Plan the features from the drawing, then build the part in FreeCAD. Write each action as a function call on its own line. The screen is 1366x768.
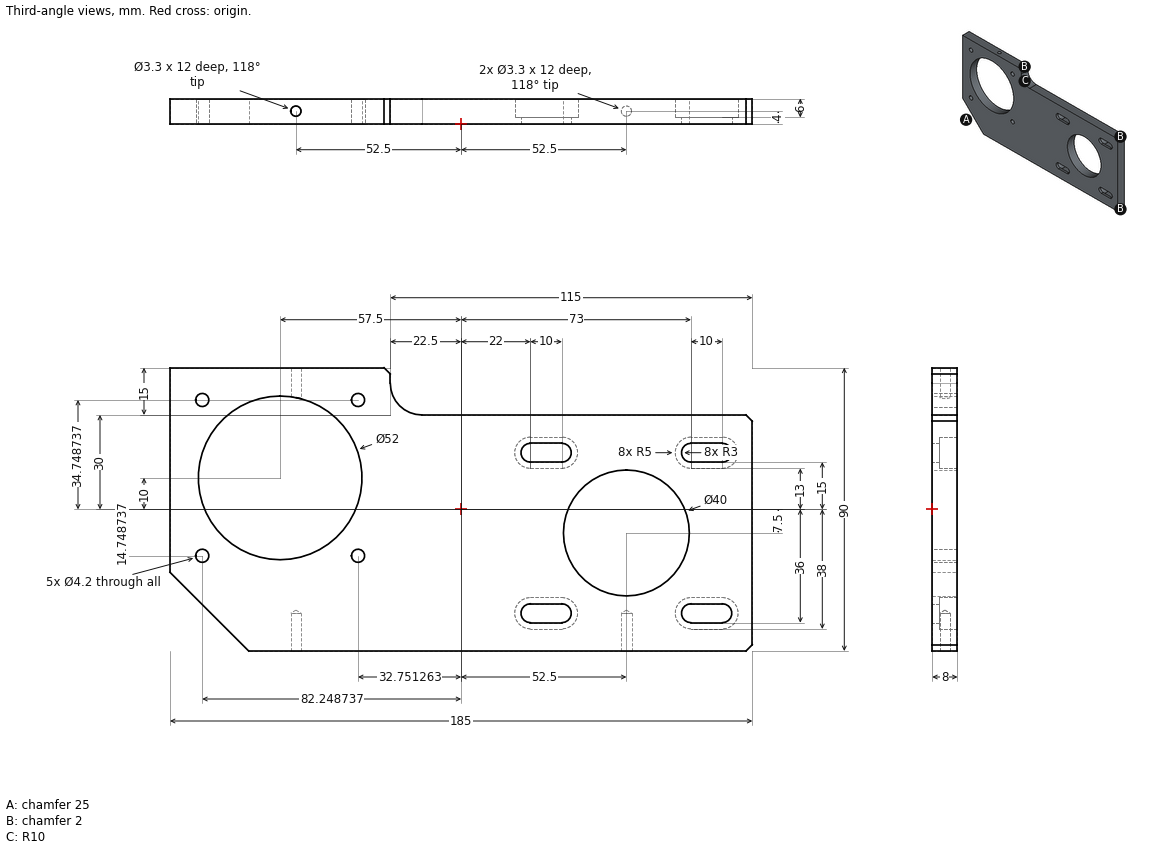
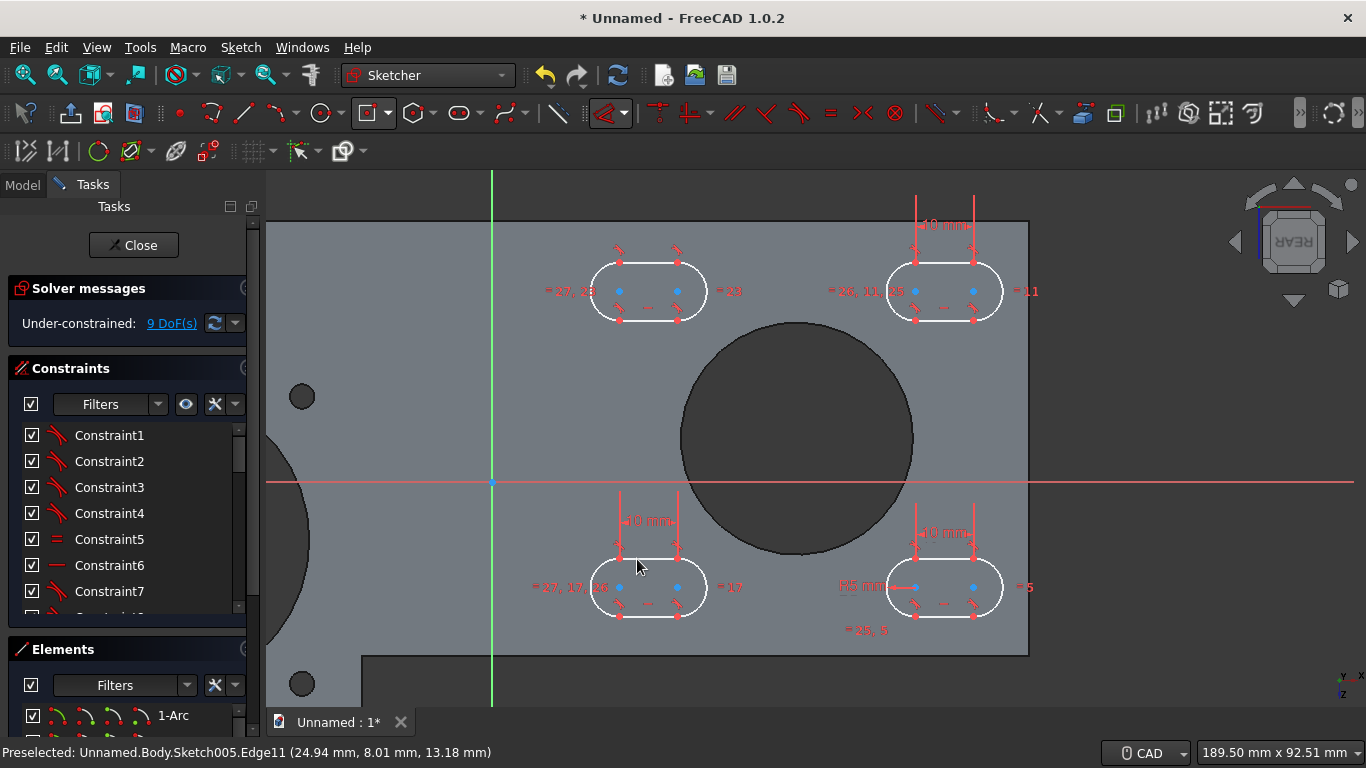
click(637, 263)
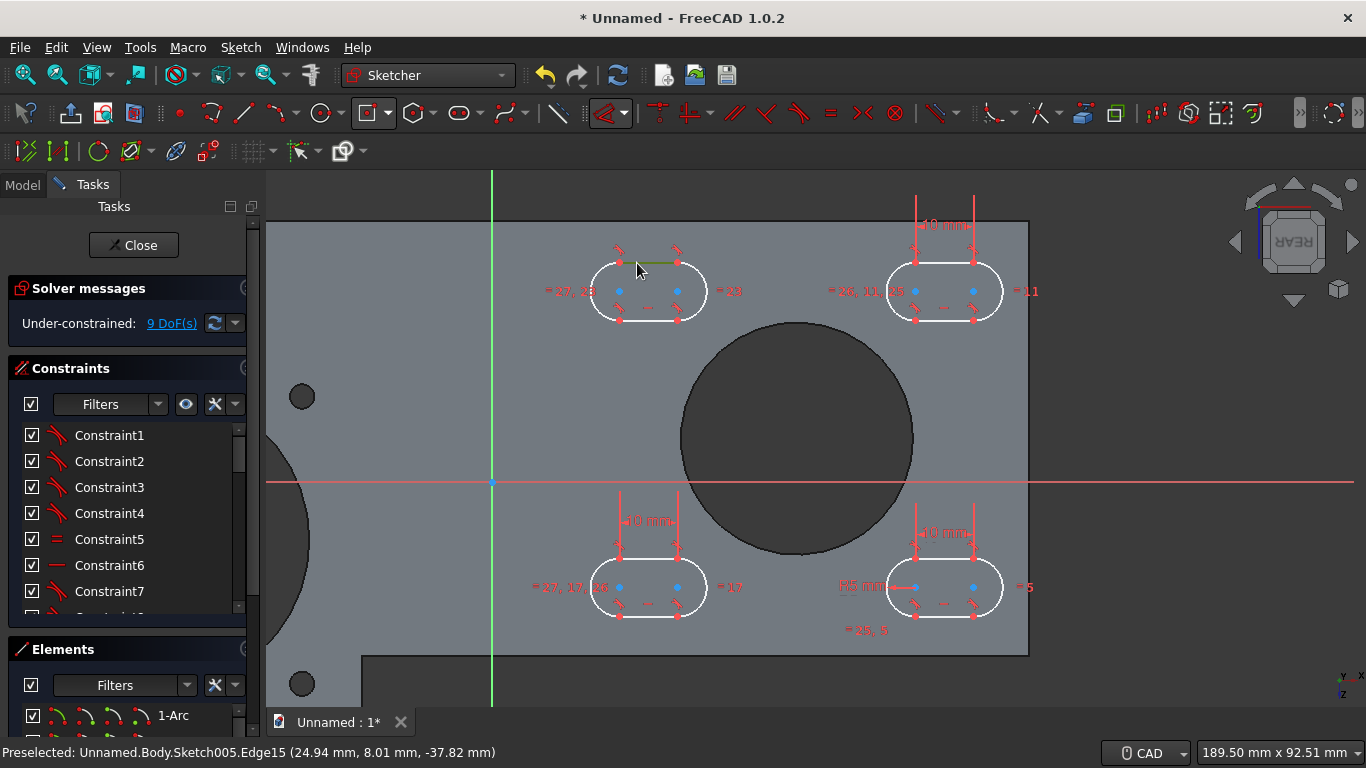
click(626, 114)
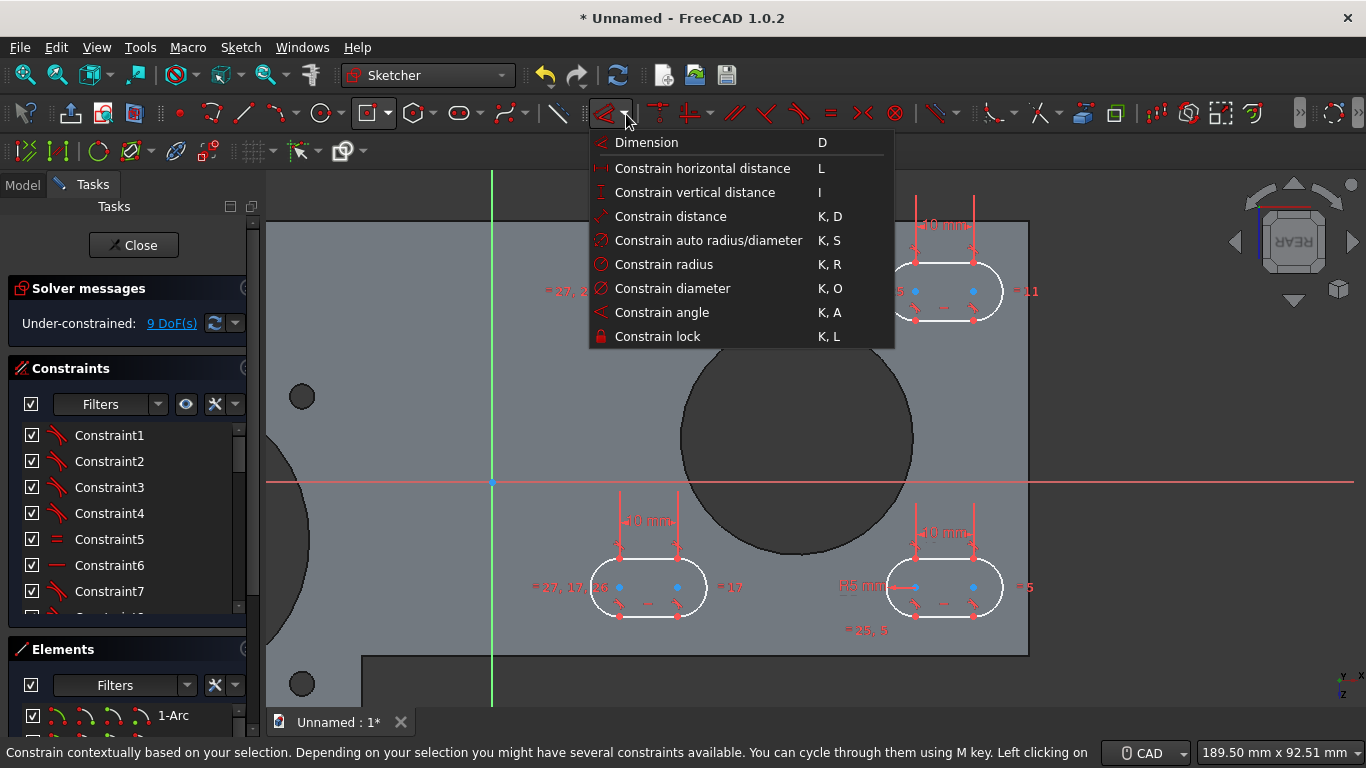
click(742, 168)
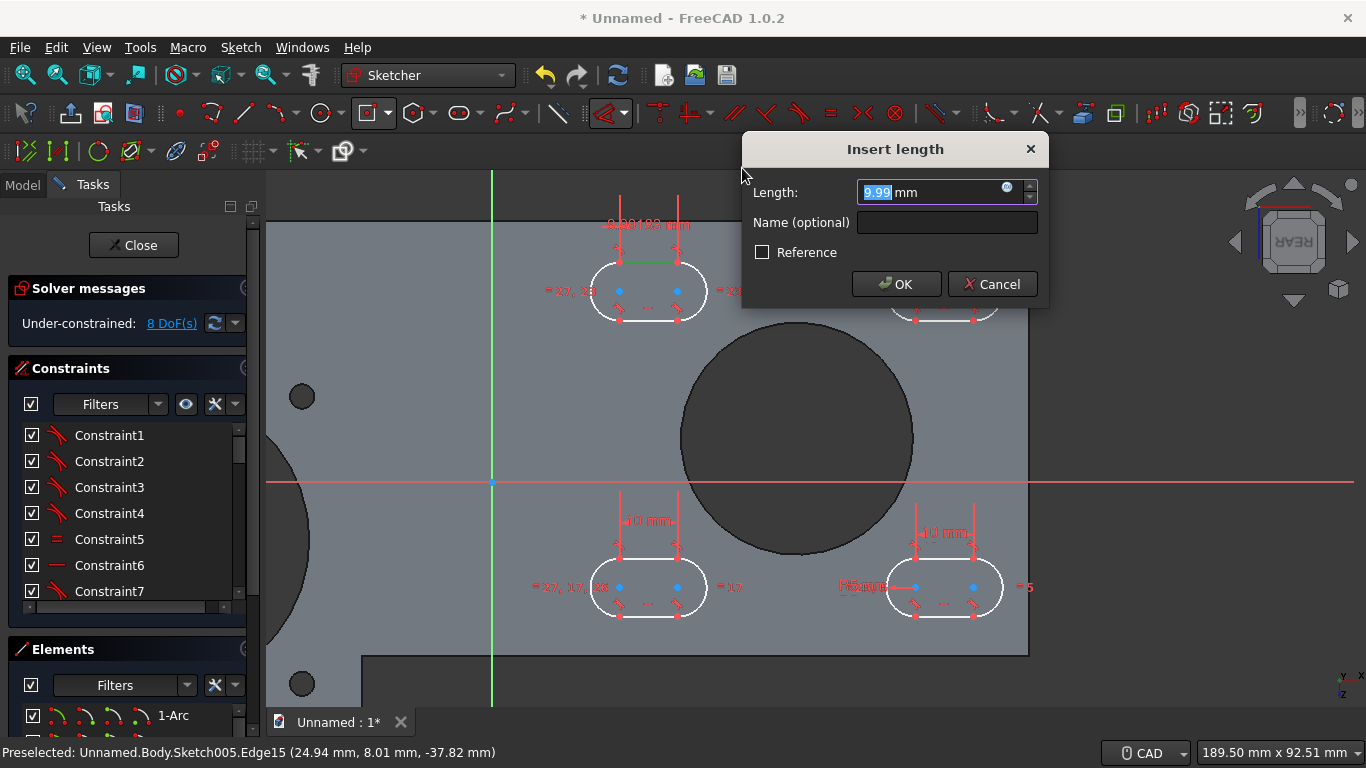
text(10)
key(Return)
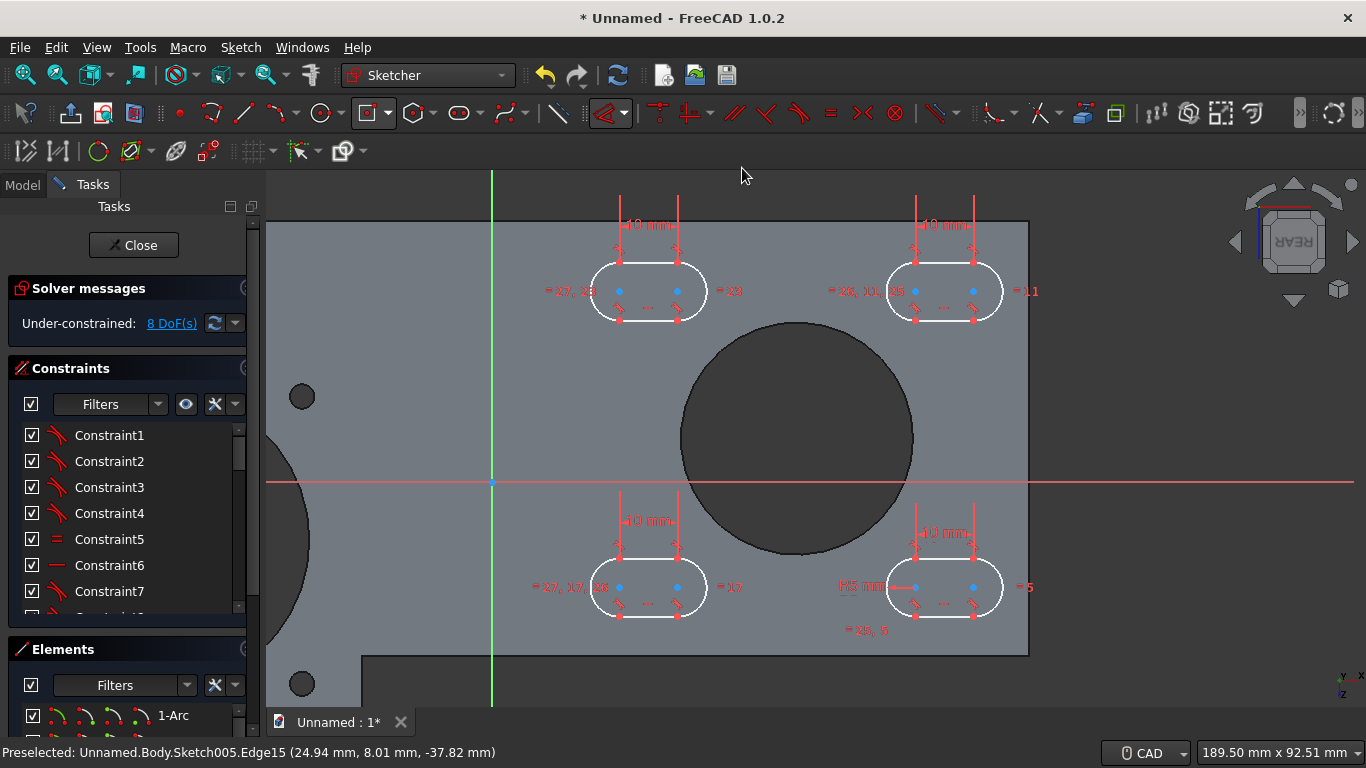
click(916, 559)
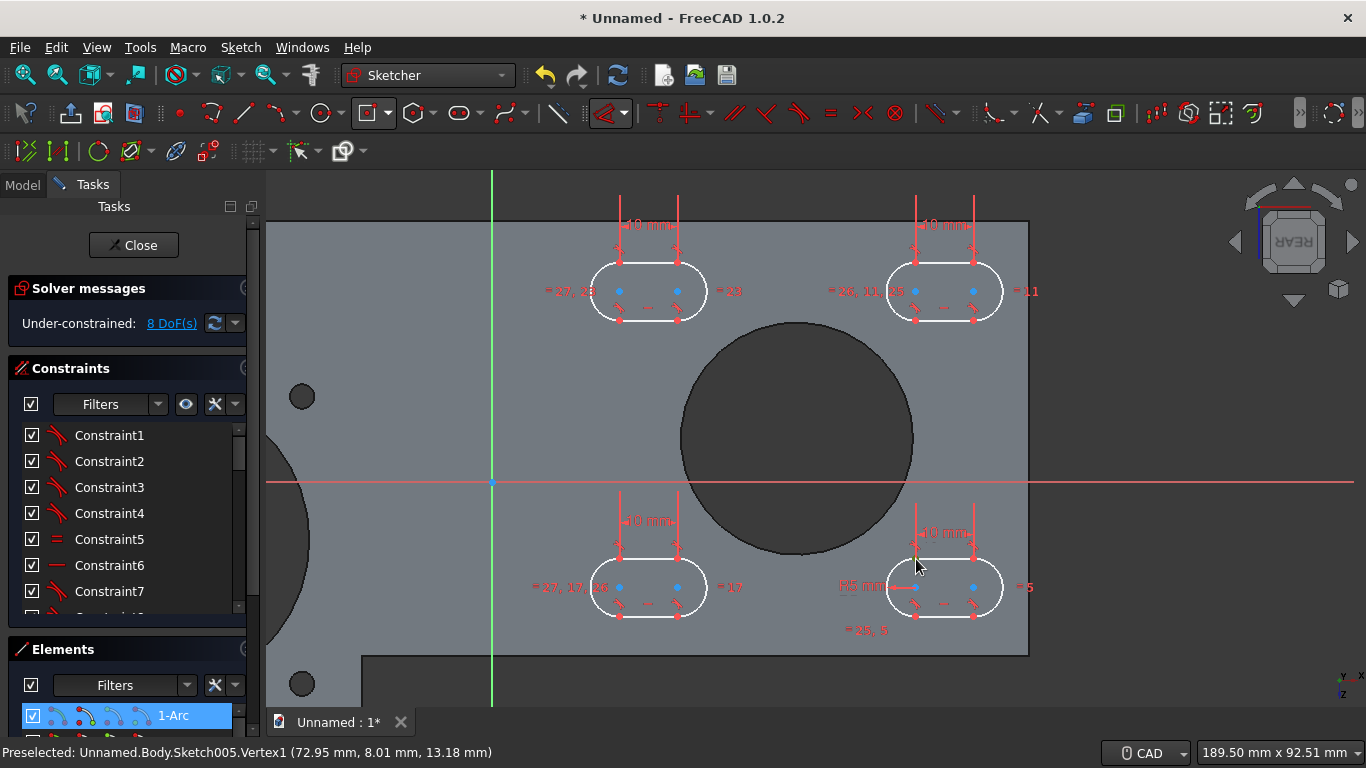
key(l)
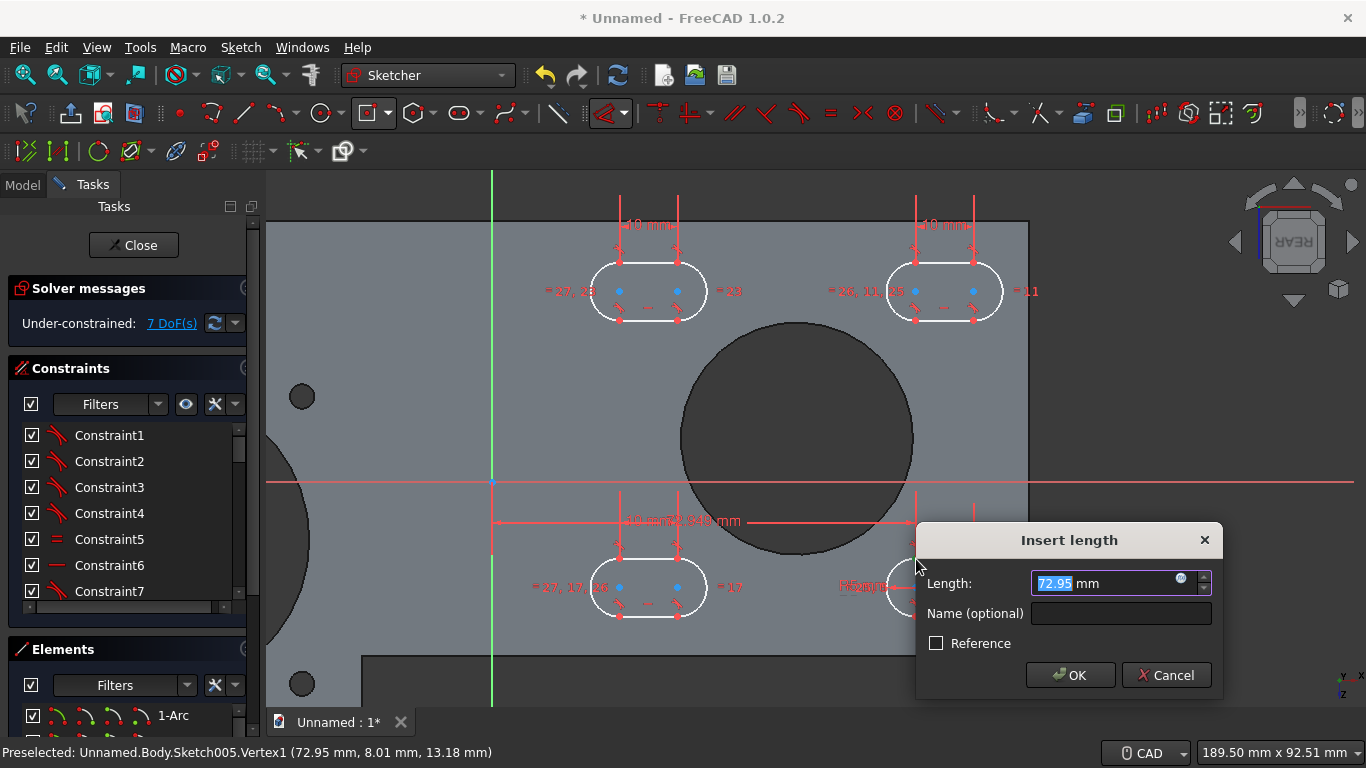
text(73)
key(Return)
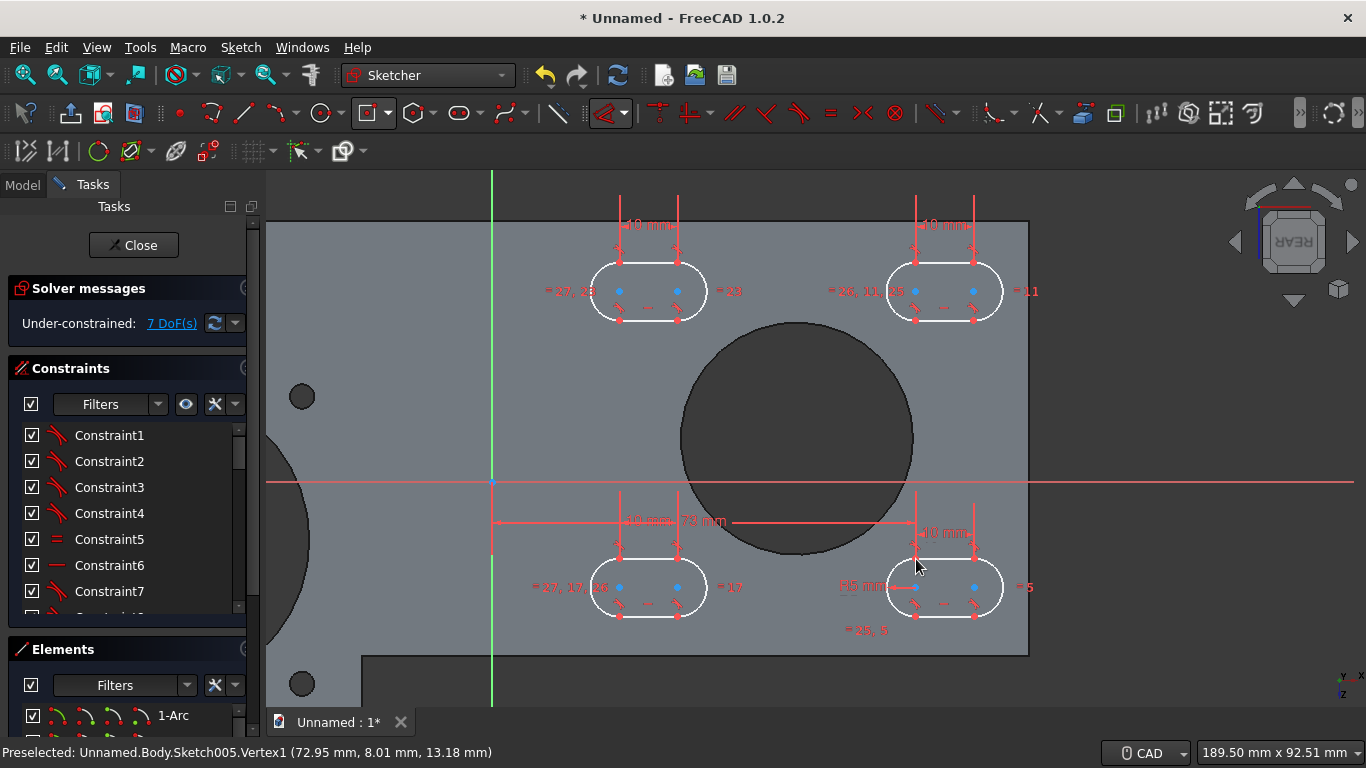
click(916, 559)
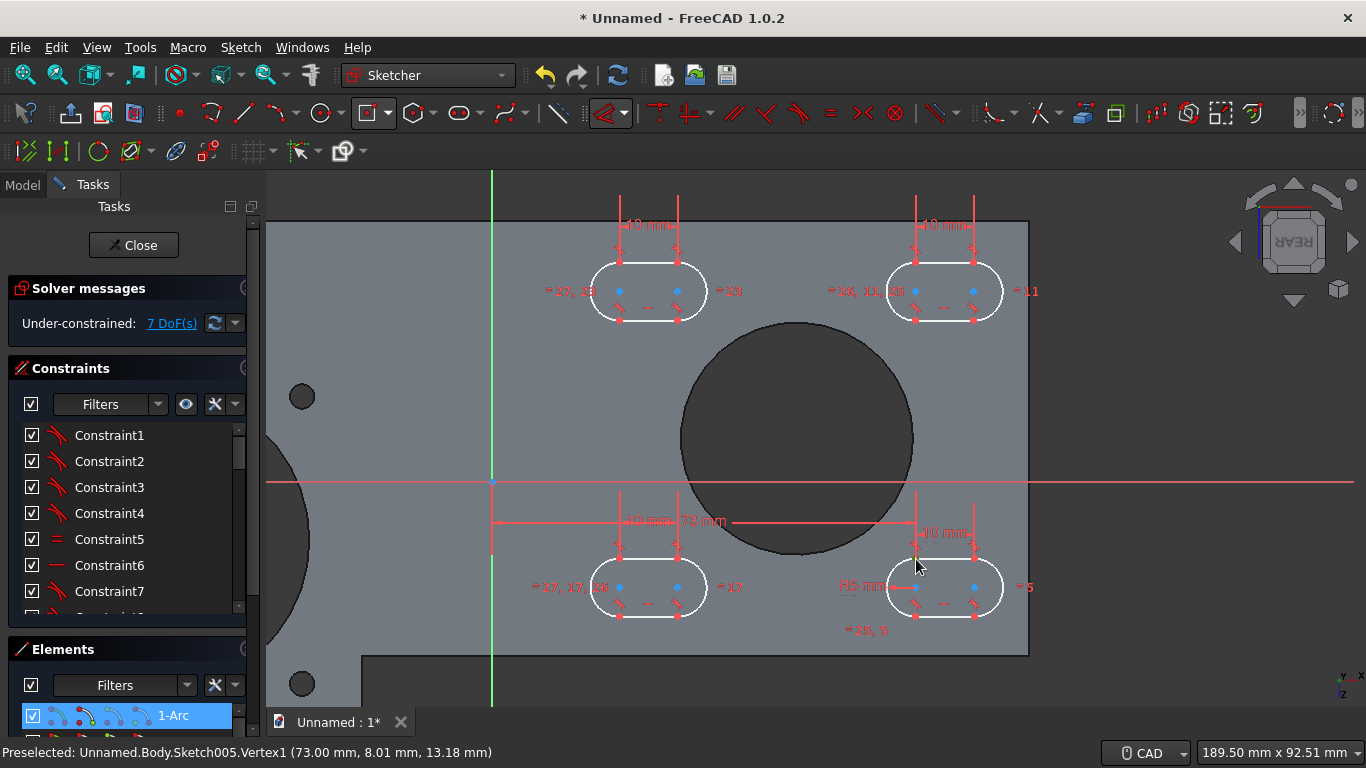
key(i)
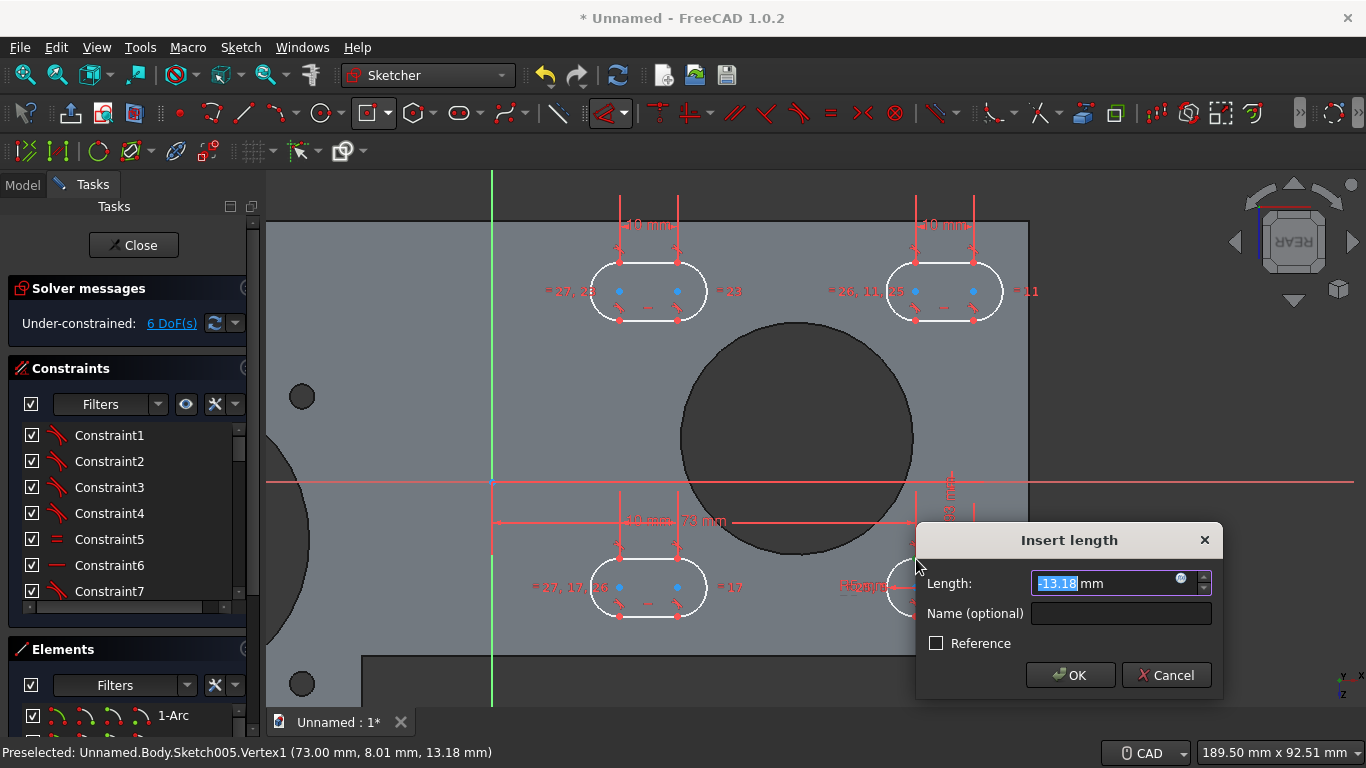
text(-13)
key(Return)